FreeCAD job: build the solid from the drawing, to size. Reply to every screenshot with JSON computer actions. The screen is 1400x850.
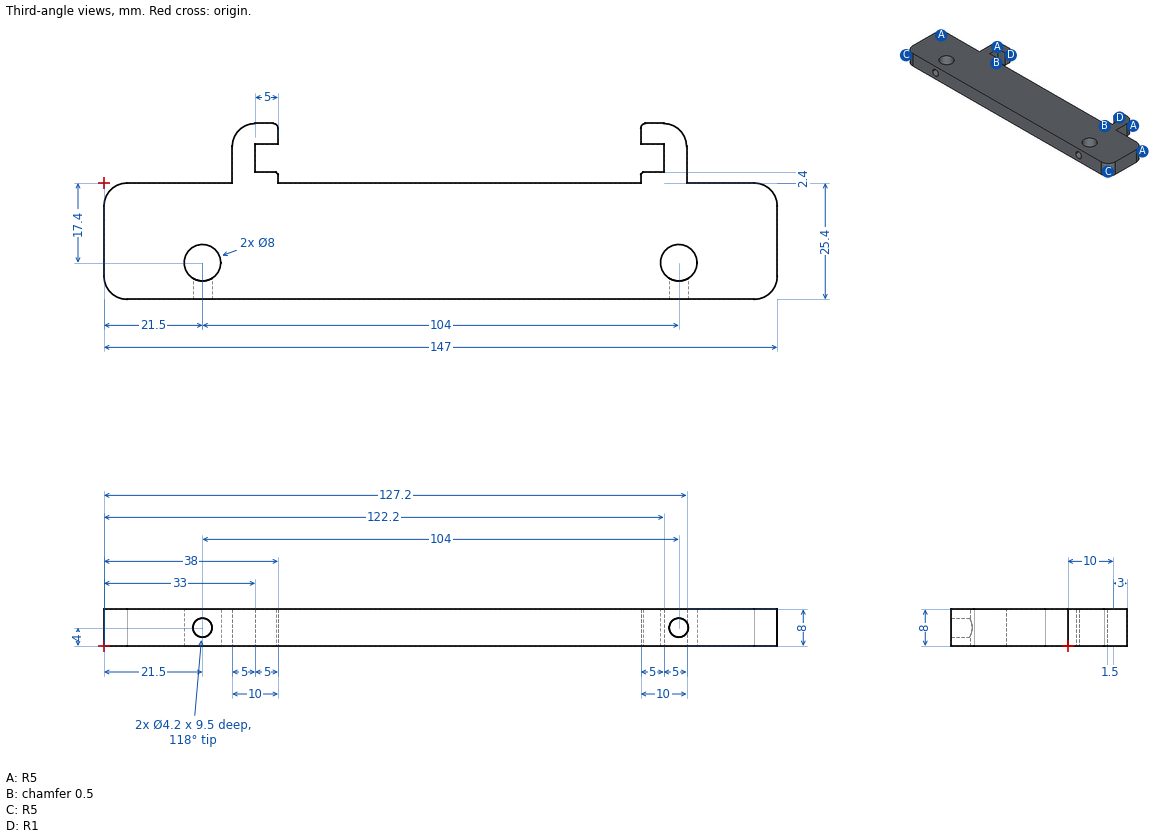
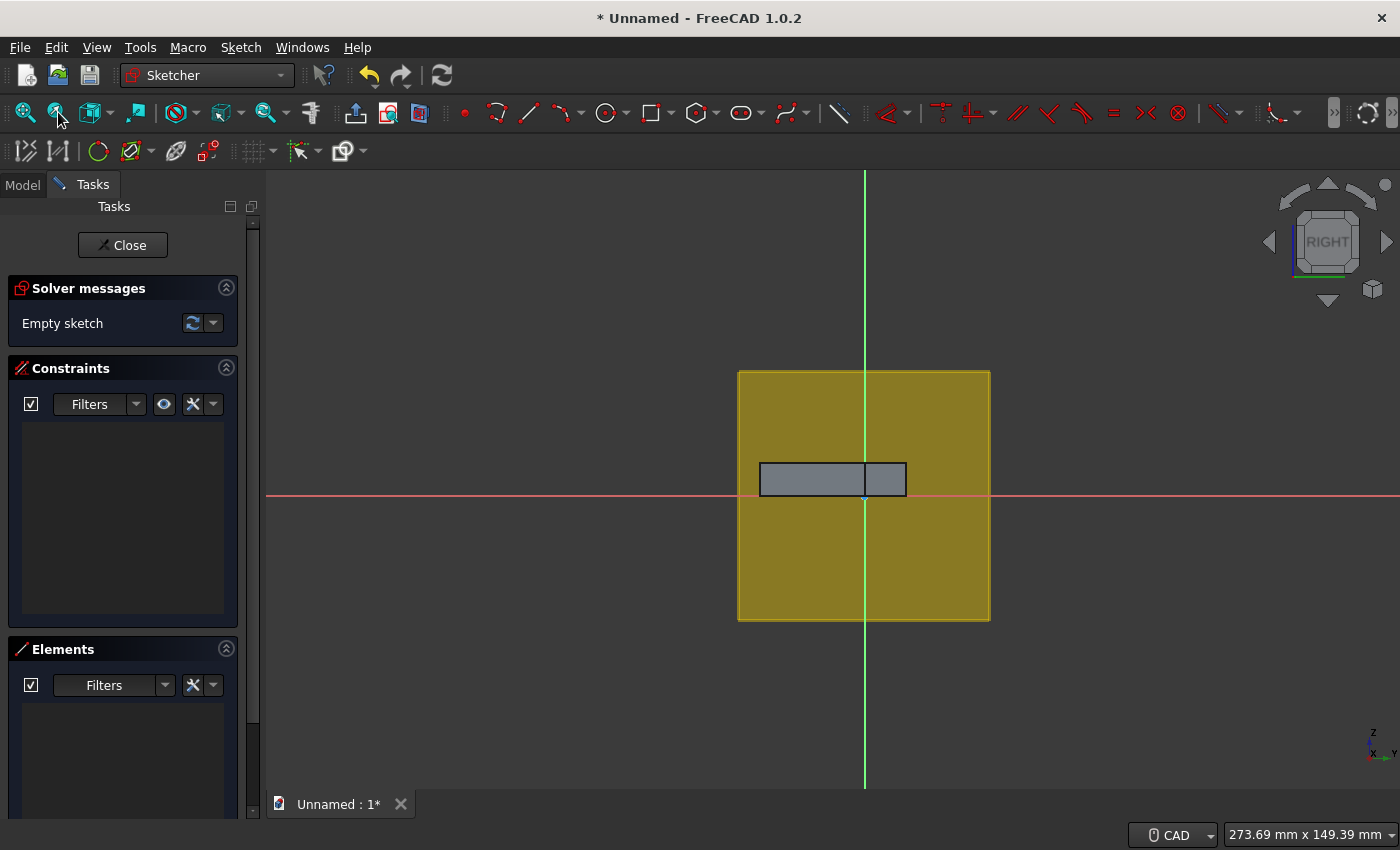
{"action": "left_click", "coordinate": [420, 114]}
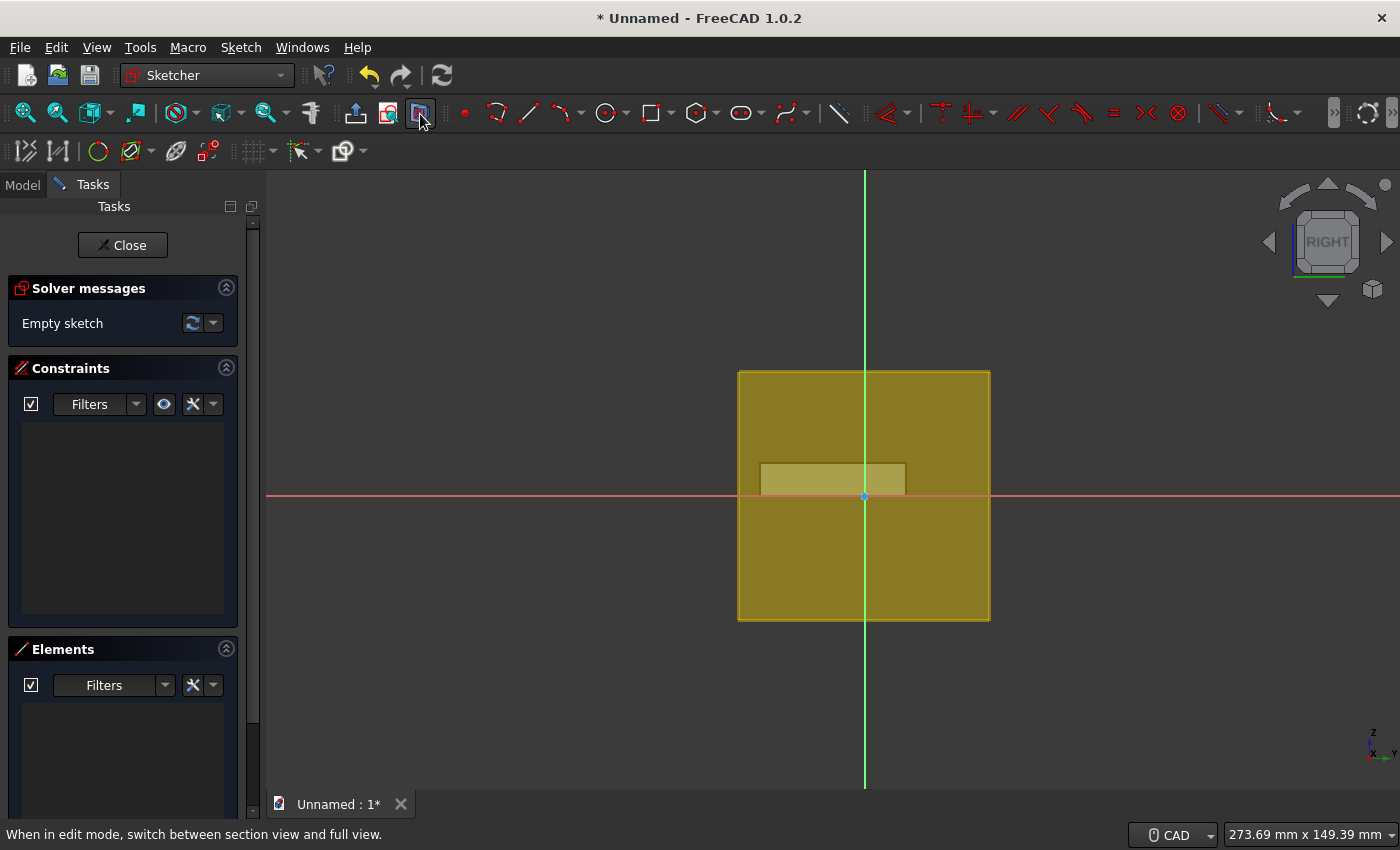
{"action": "scroll", "coordinate": [898, 480], "scroll_direction": "up", "scroll_amount": 12}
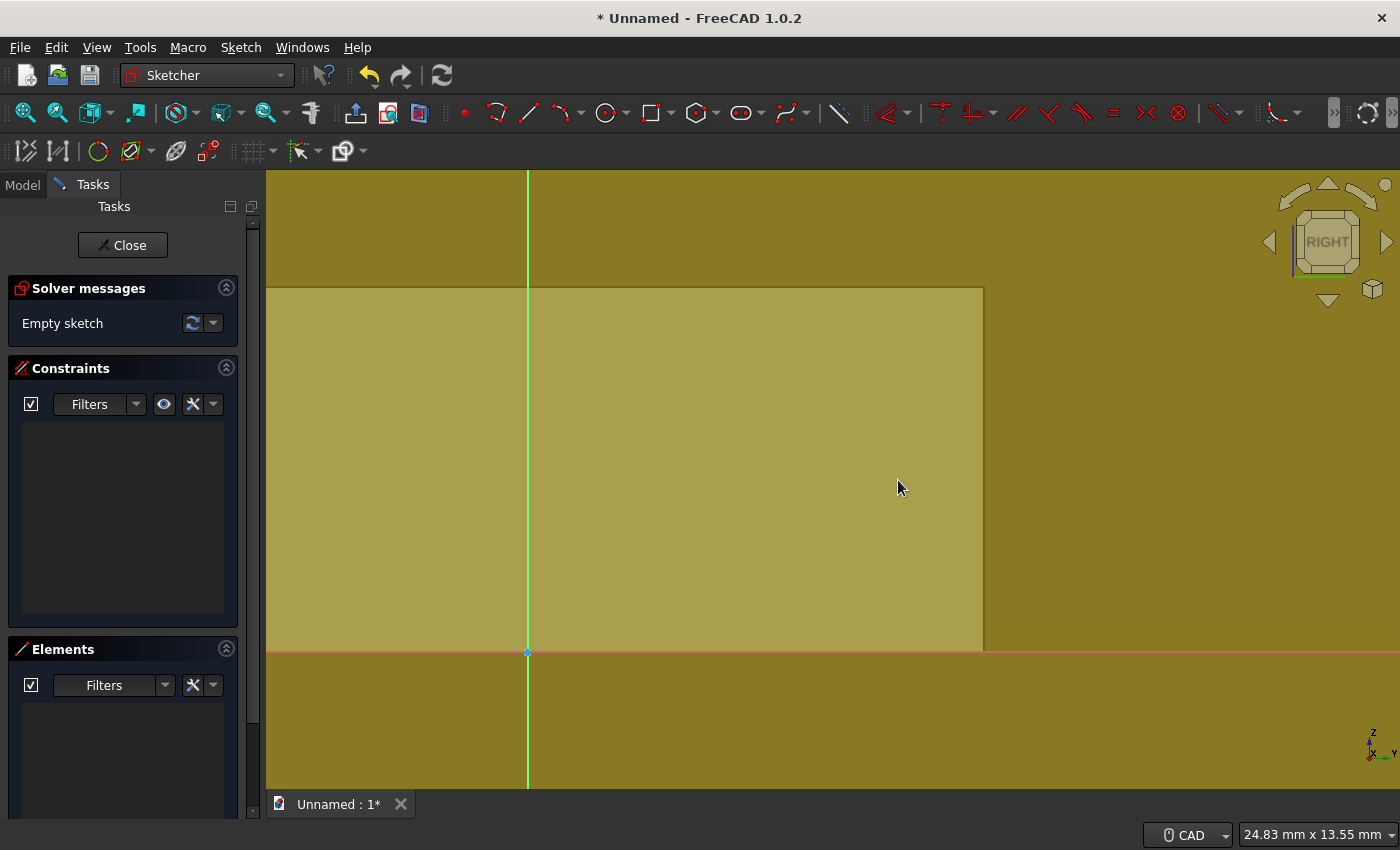
{"action": "left_click", "coordinate": [652, 114]}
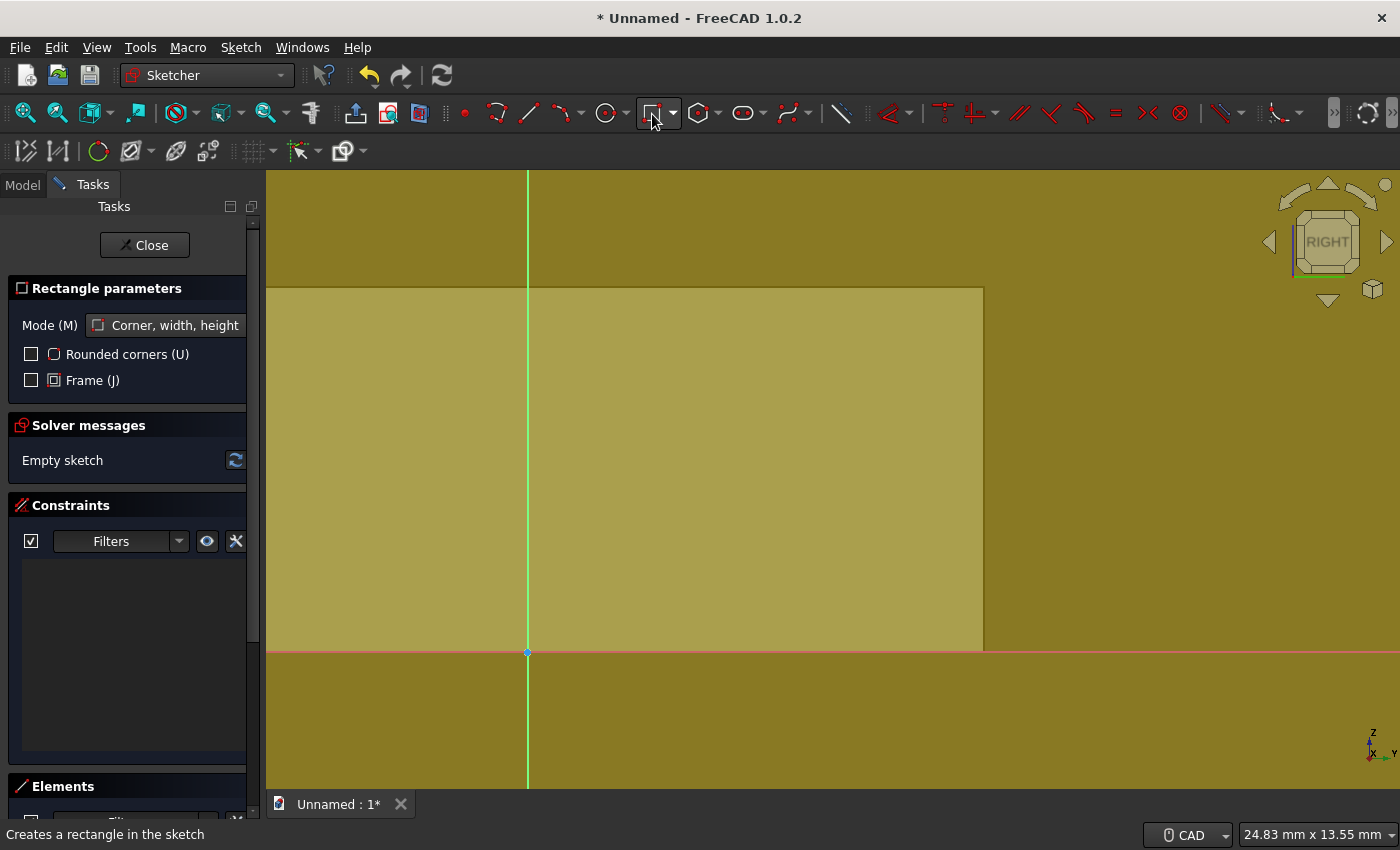
{"action": "left_click", "coordinate": [916, 287]}
{"action": "left_click", "coordinate": [984, 652]}
{"action": "key", "text": "Escape"}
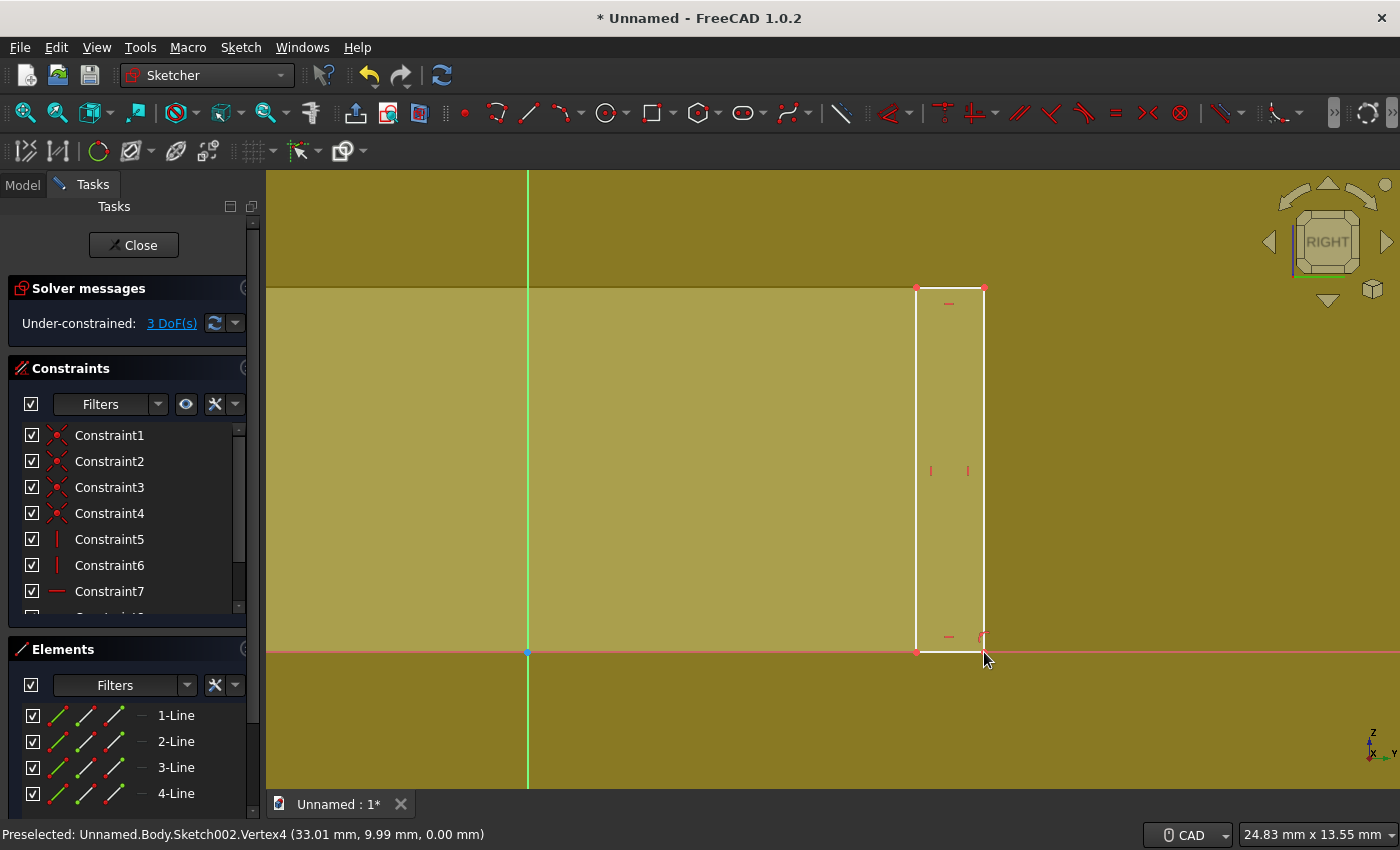
{"action": "left_click", "coordinate": [888, 114]}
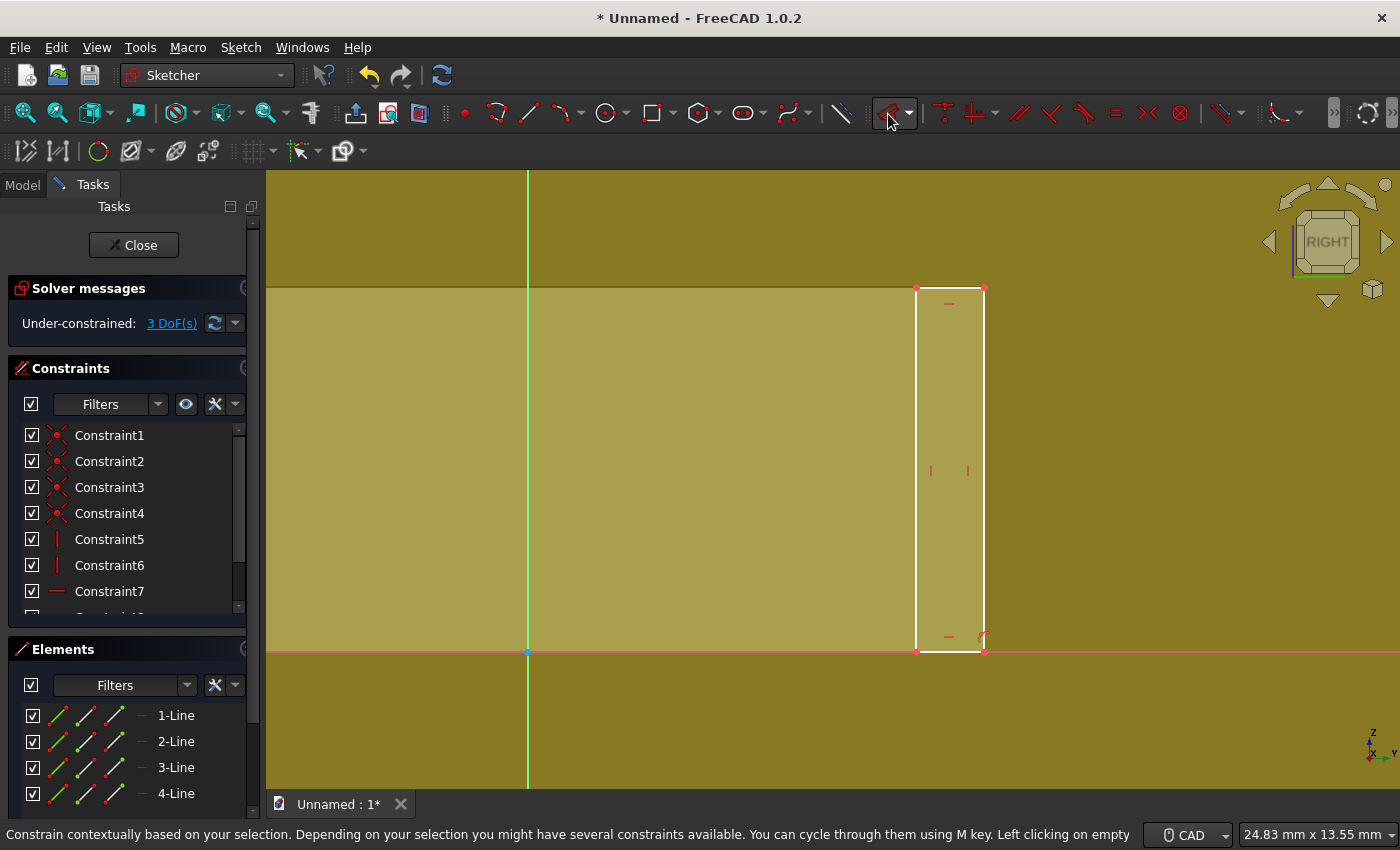
{"action": "left_click", "coordinate": [916, 397]}
{"action": "left_click", "coordinate": [950, 470]}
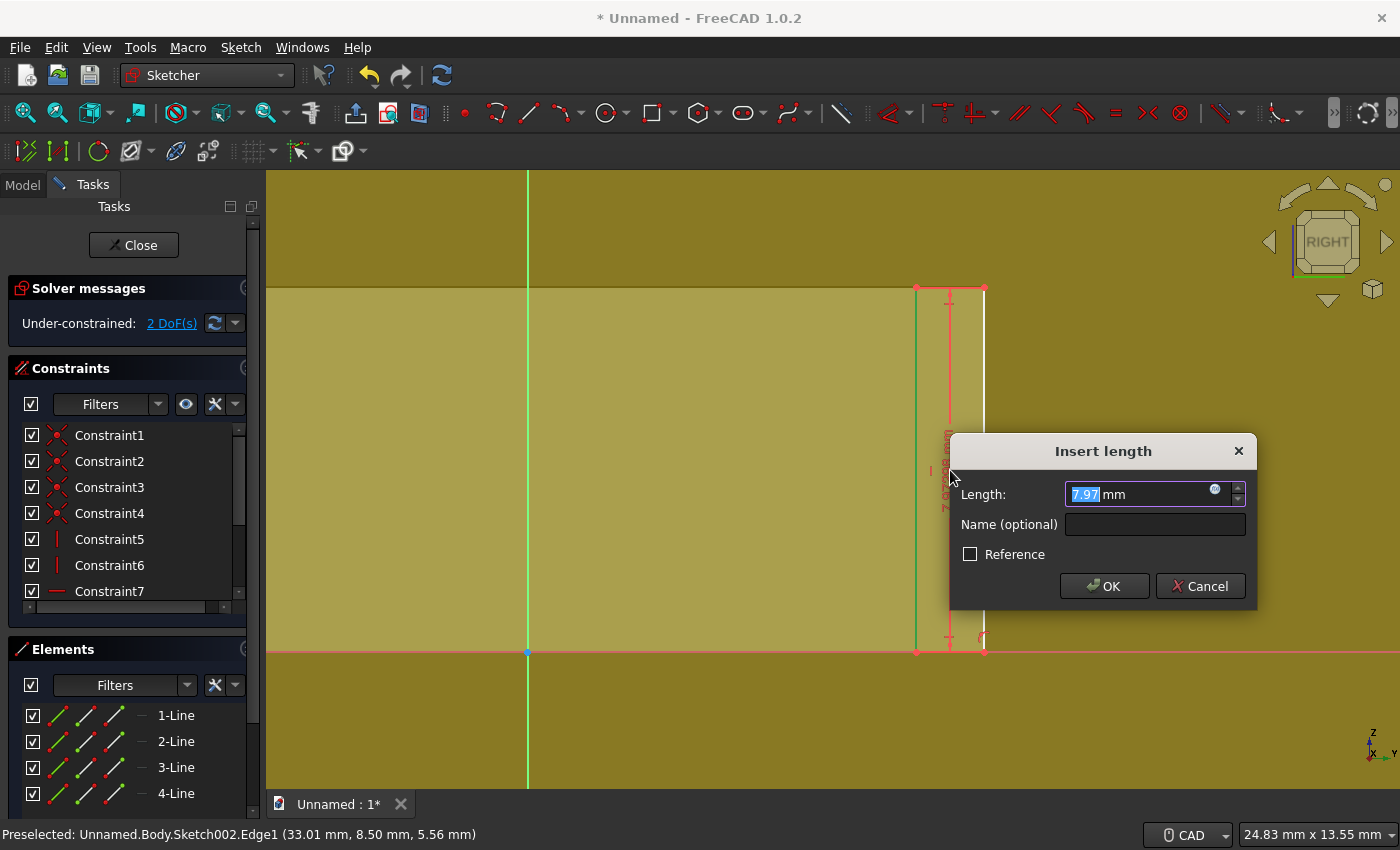
{"action": "type", "text": "8"}
{"action": "key", "text": "Return"}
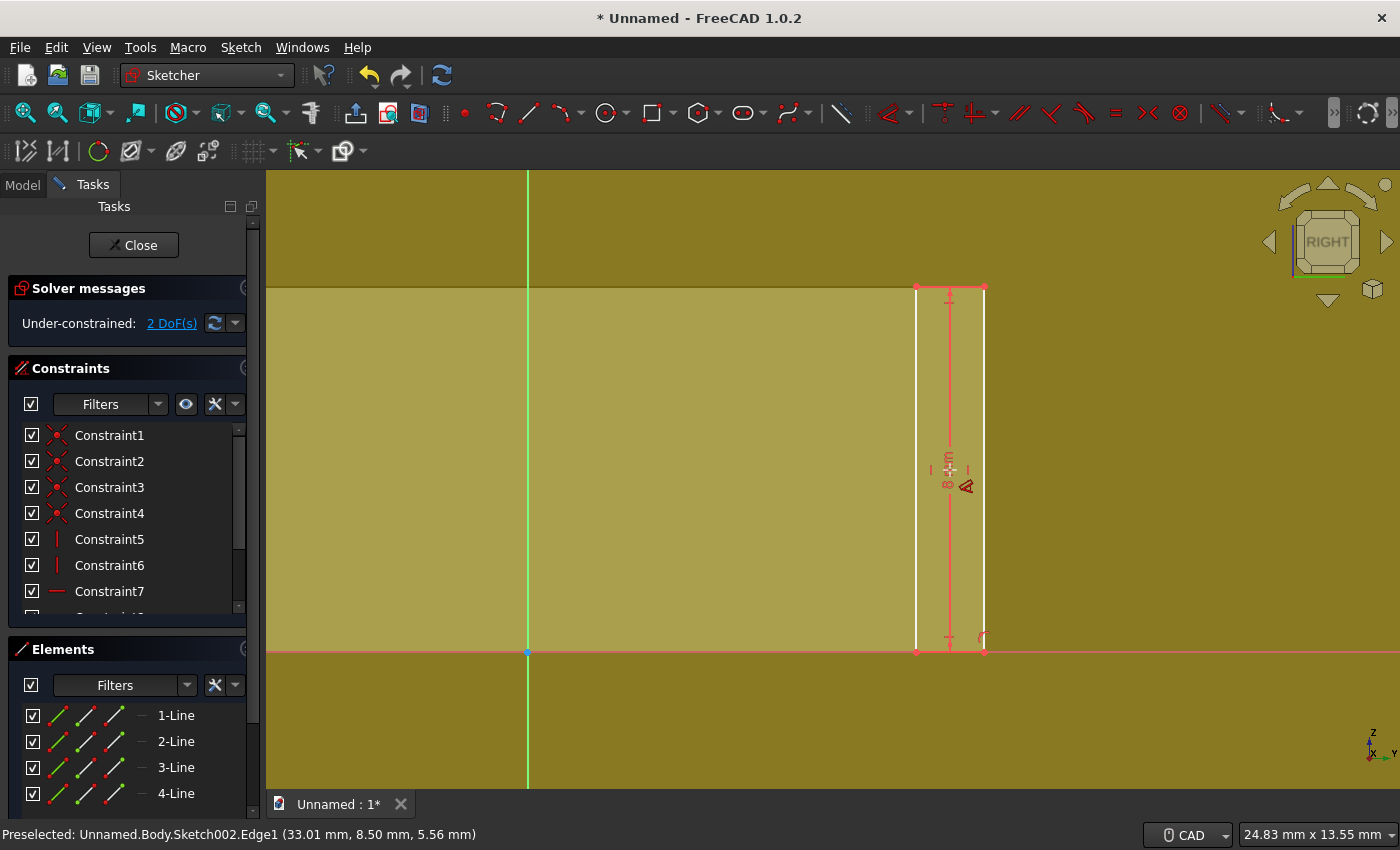
{"action": "left_click", "coordinate": [936, 652]}
{"action": "left_click", "coordinate": [950, 686]}